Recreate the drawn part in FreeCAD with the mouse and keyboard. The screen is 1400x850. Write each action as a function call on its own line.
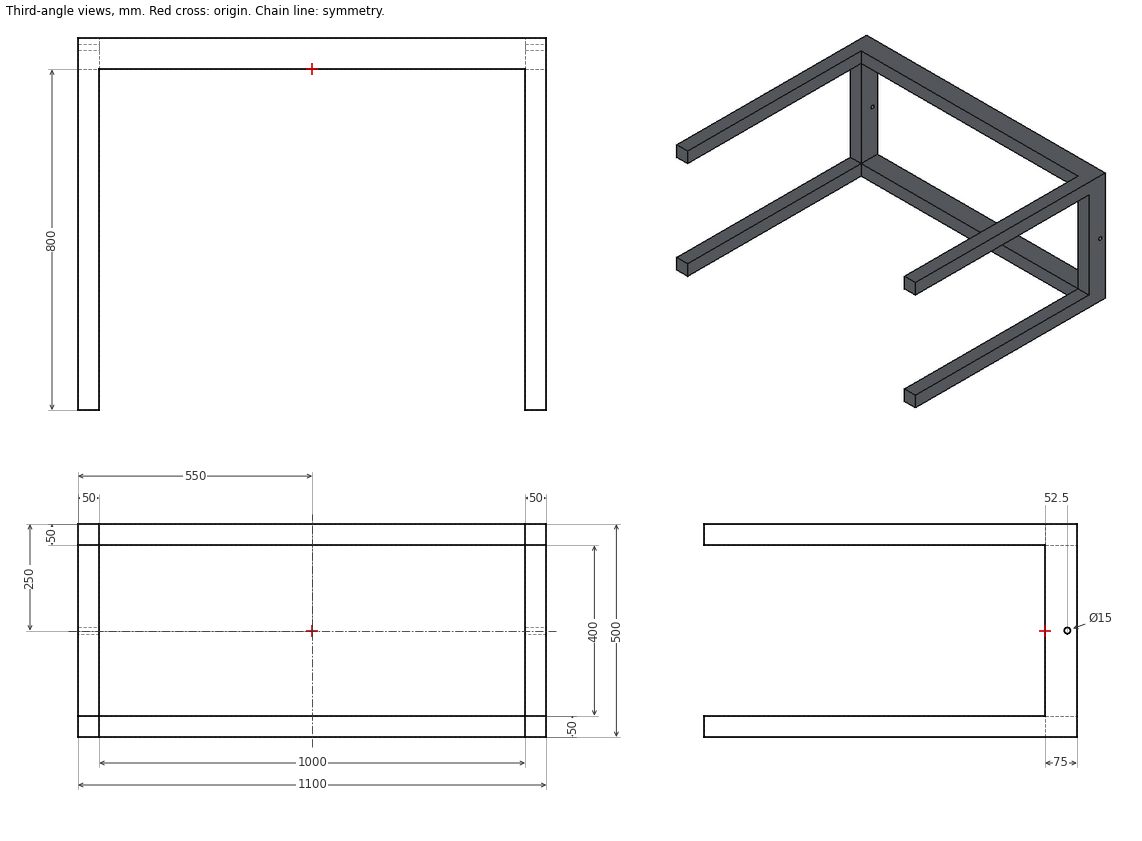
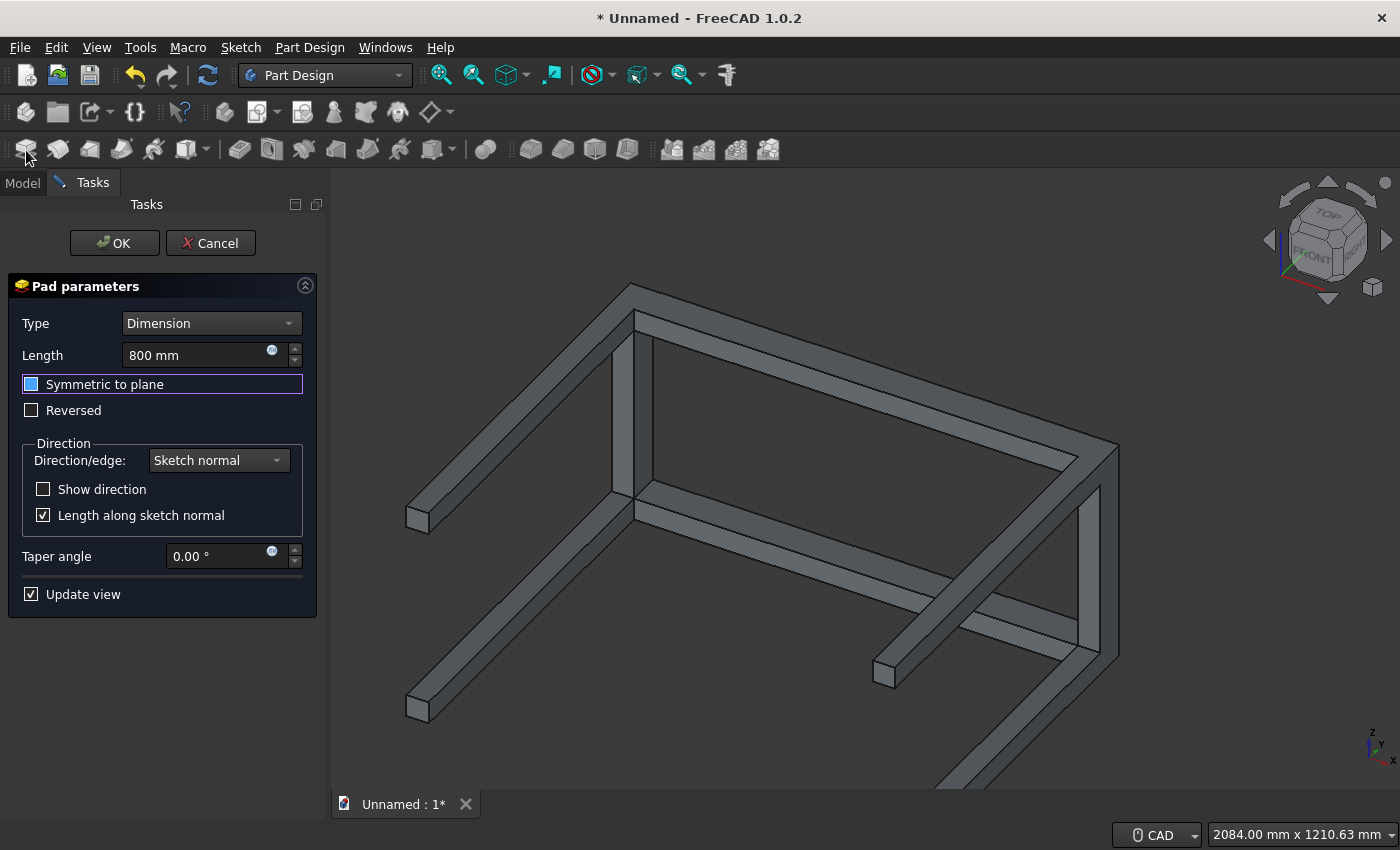
click(115, 243)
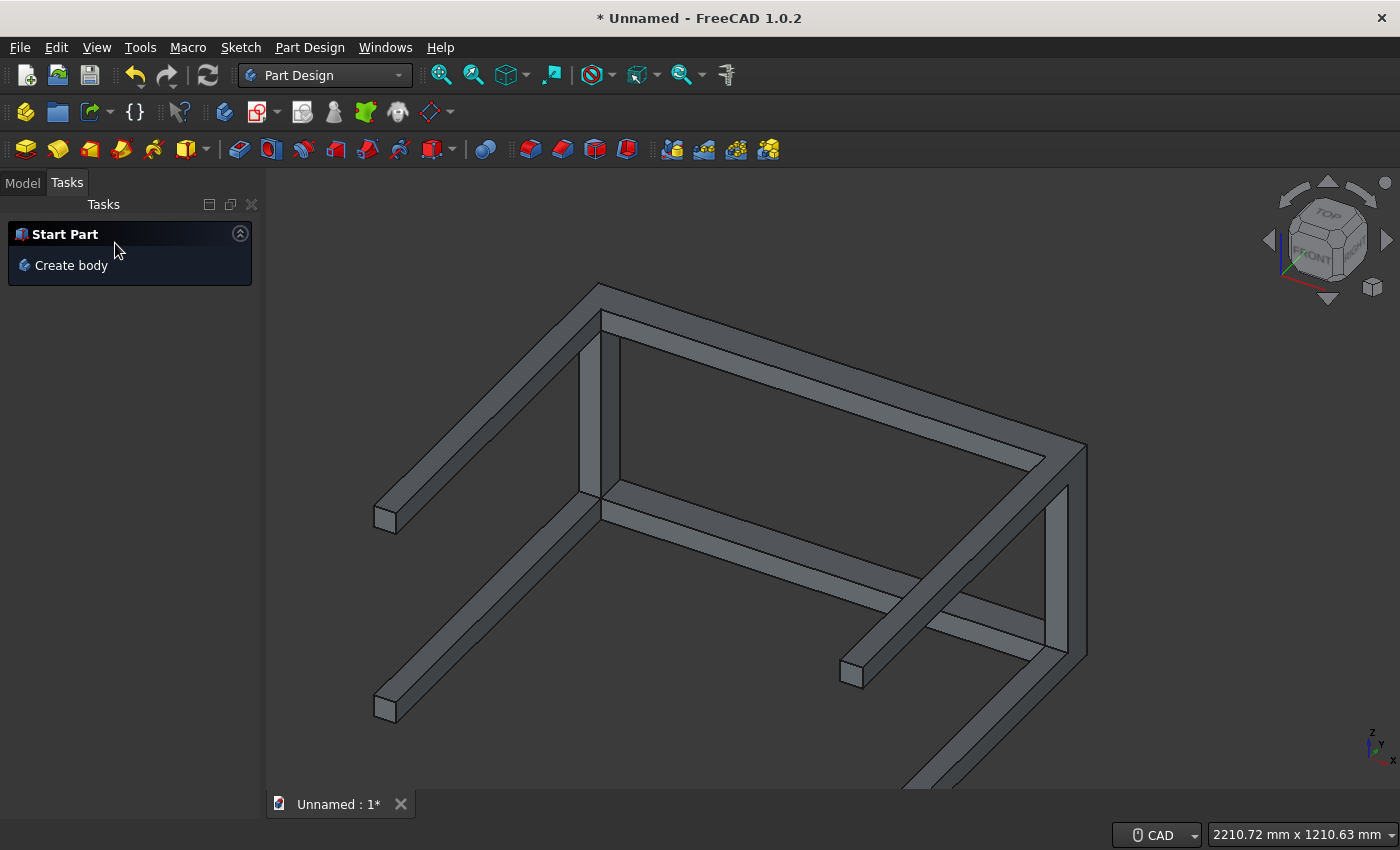
click(442, 76)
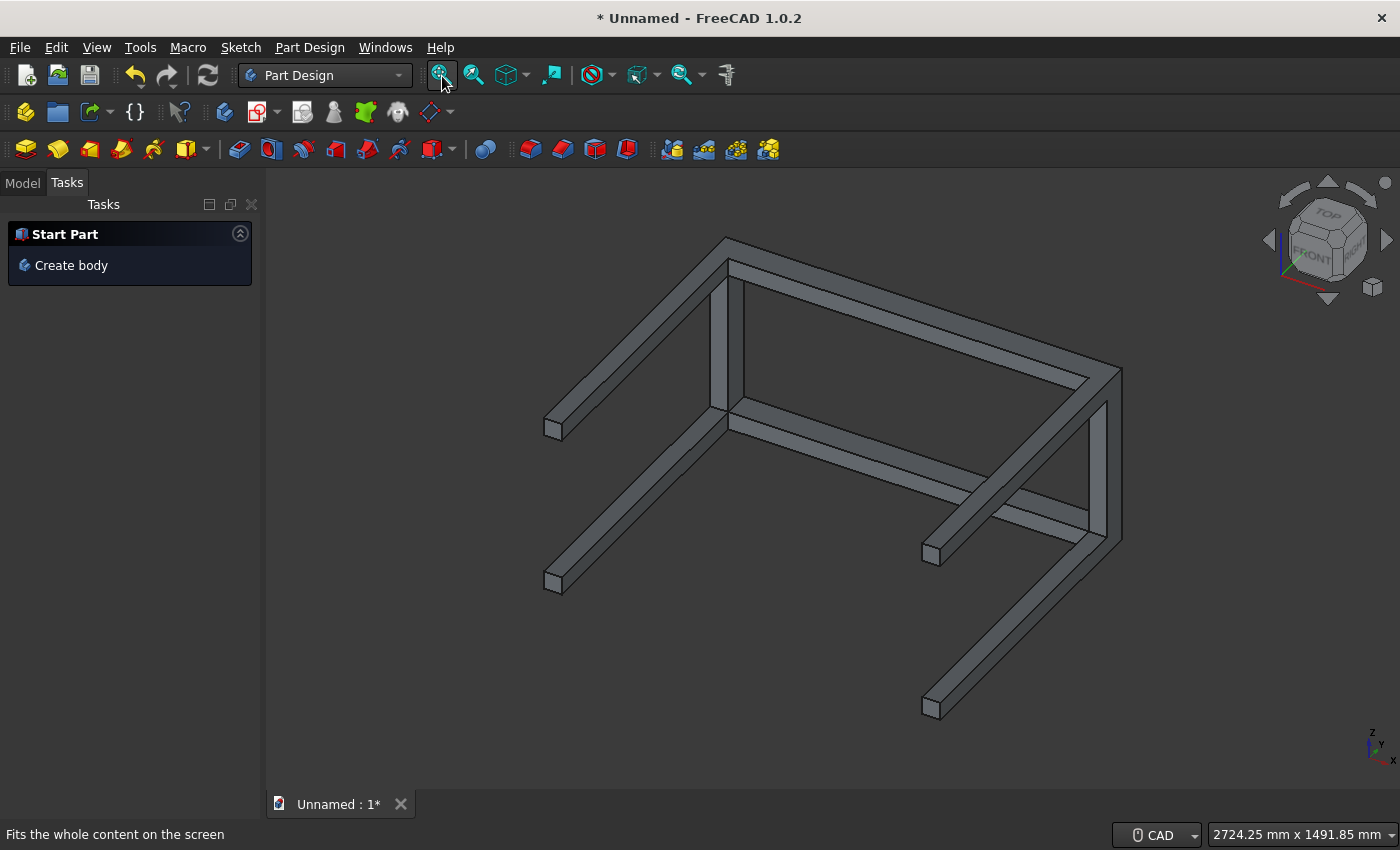
key(6)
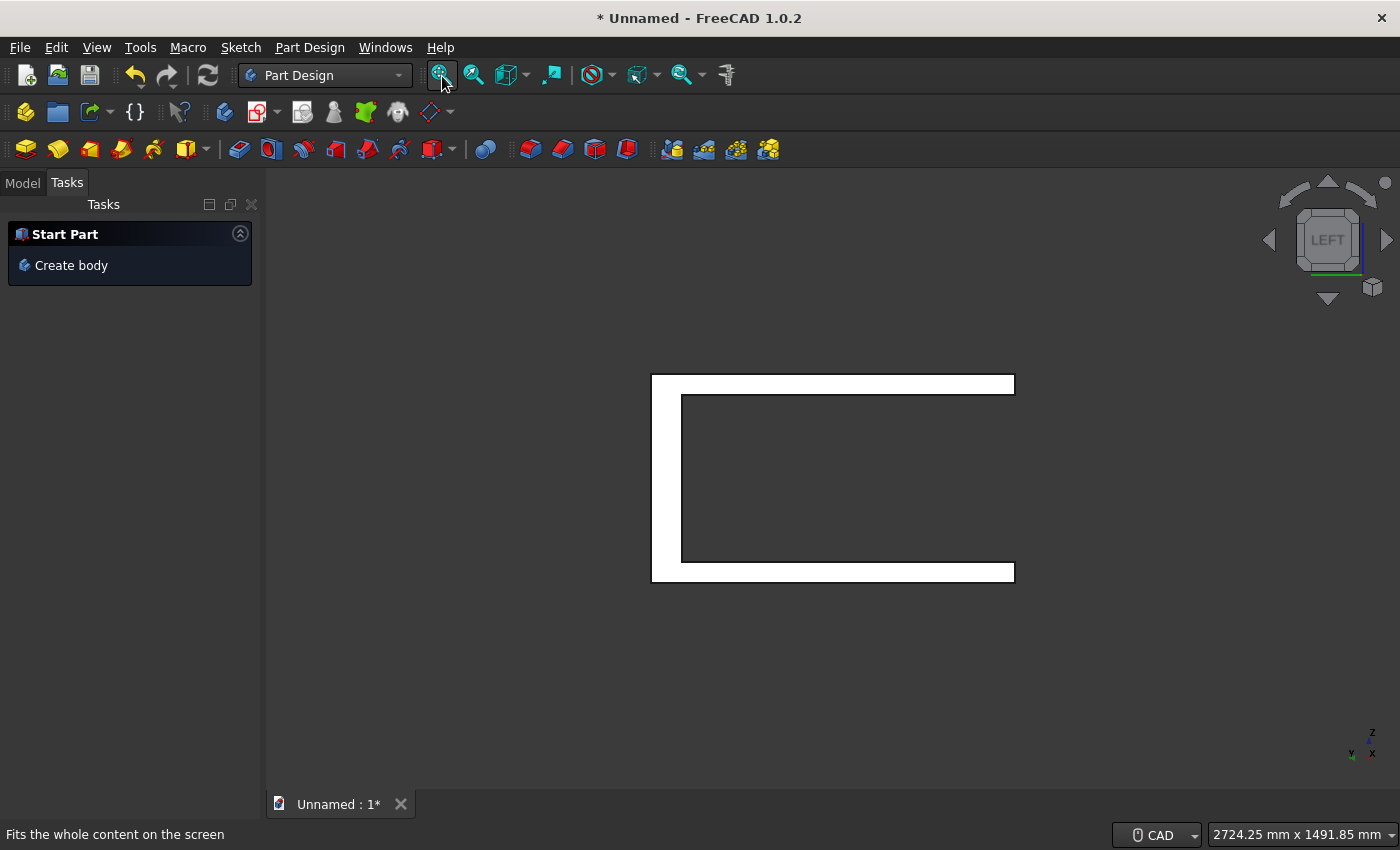
key(v)
key(f)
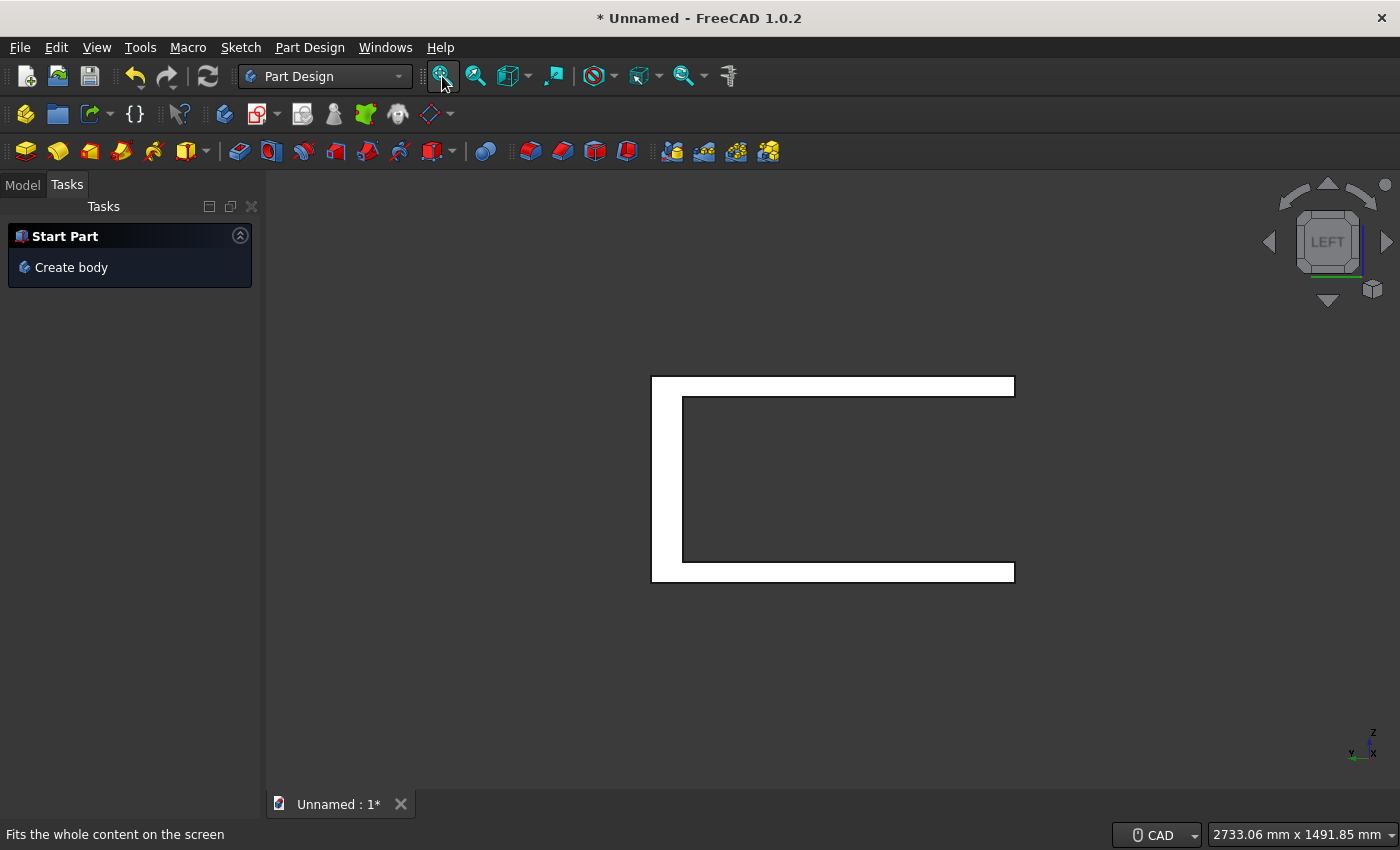
key(2)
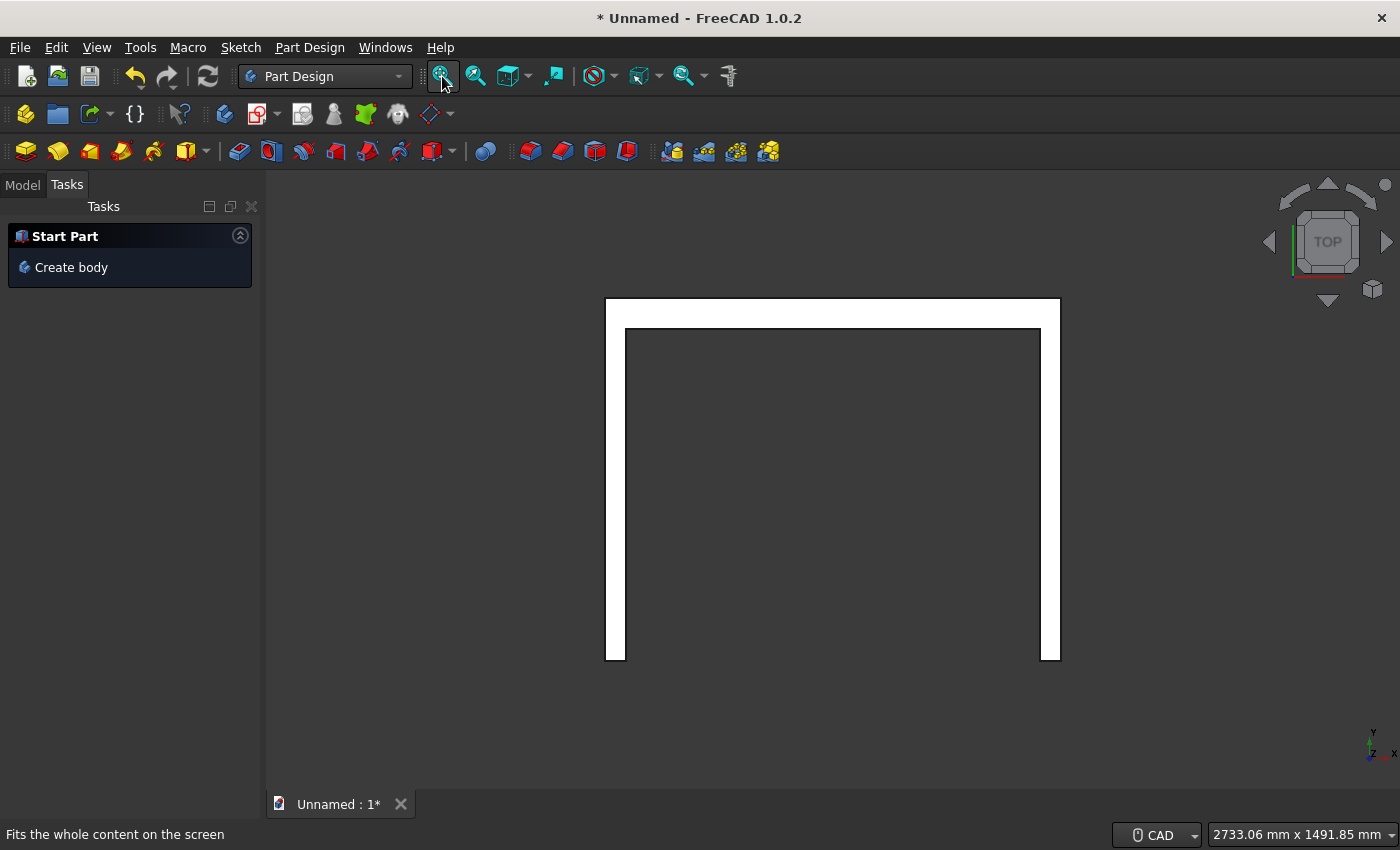
key(1)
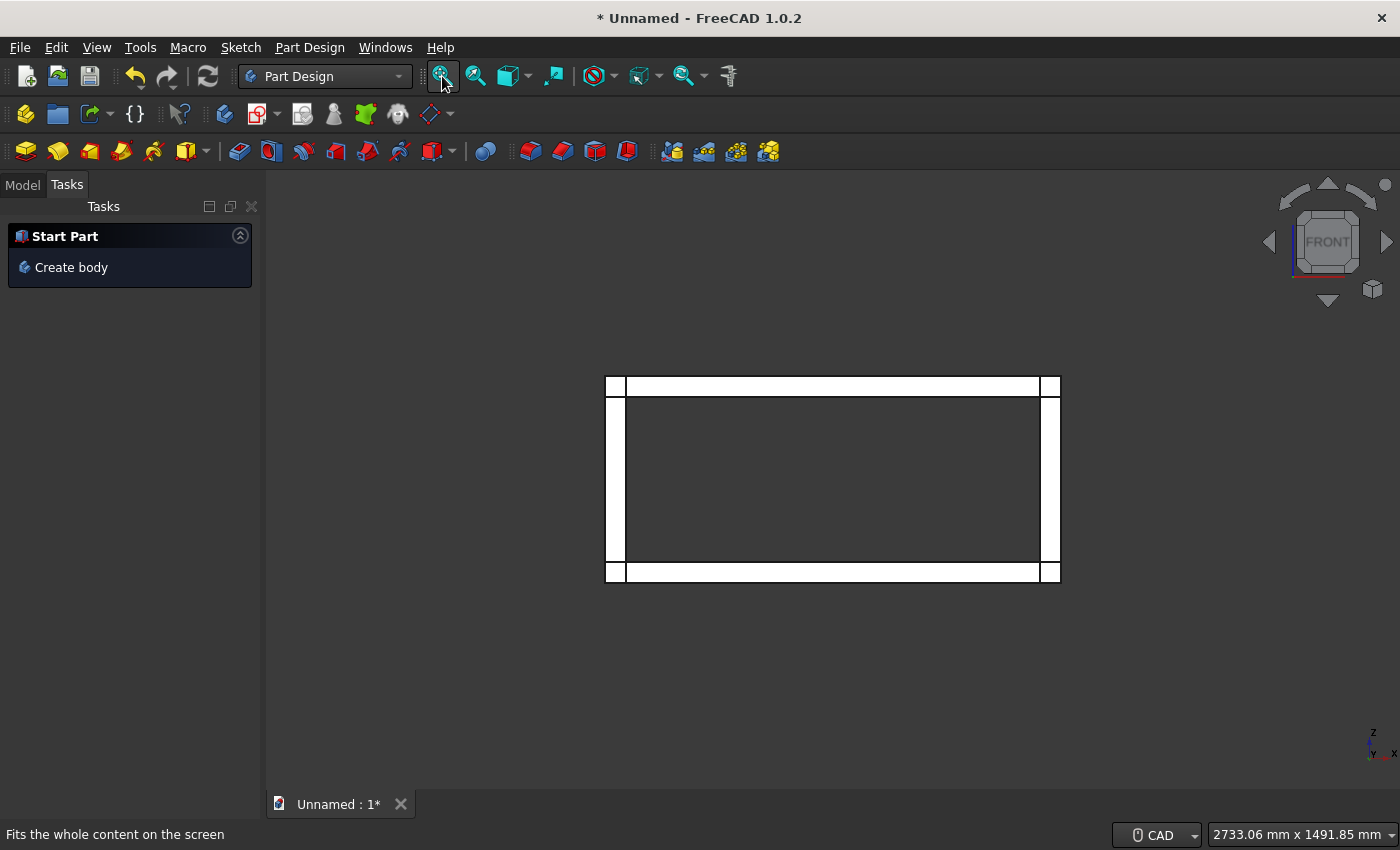
click(444, 76)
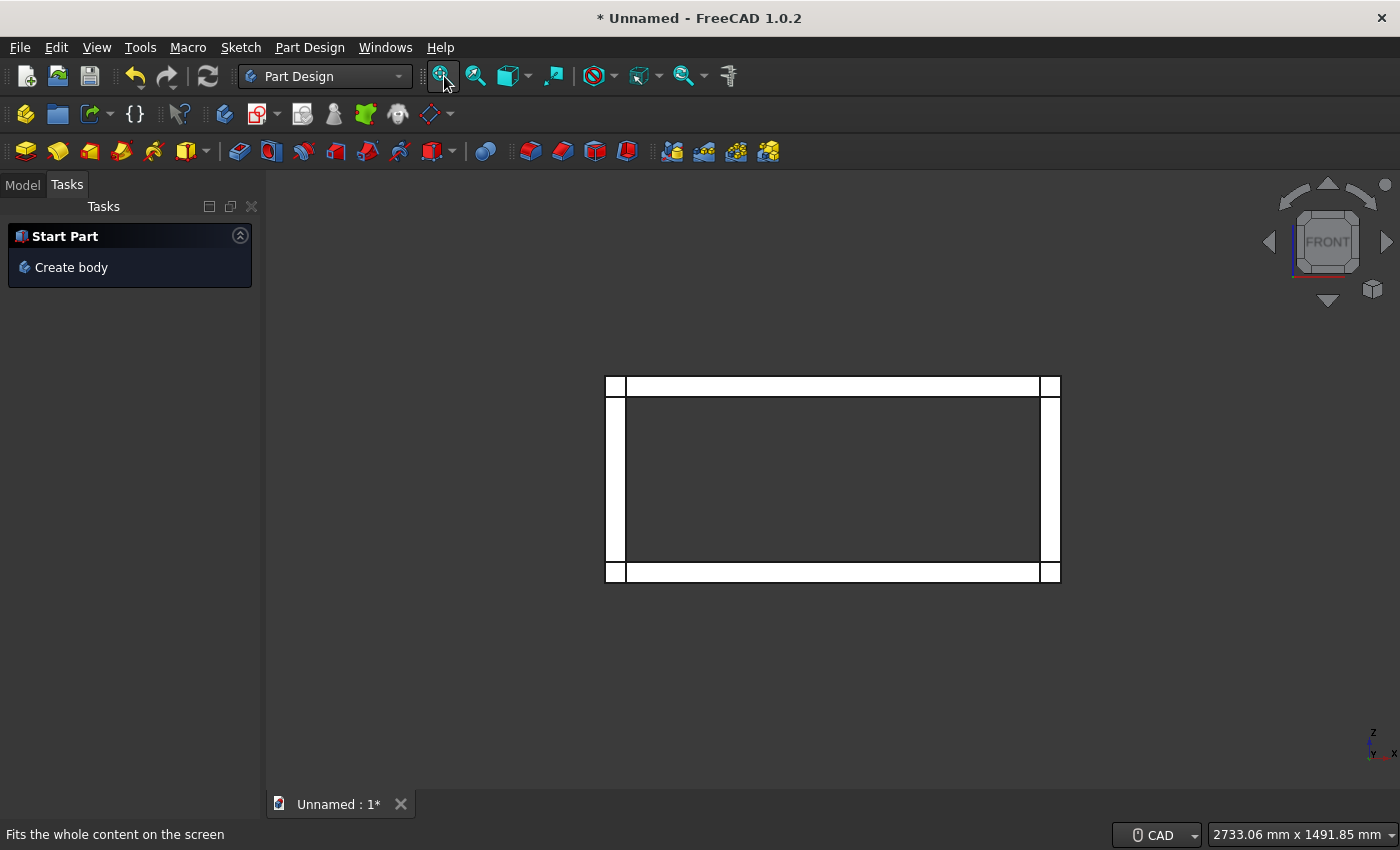
click(23, 184)